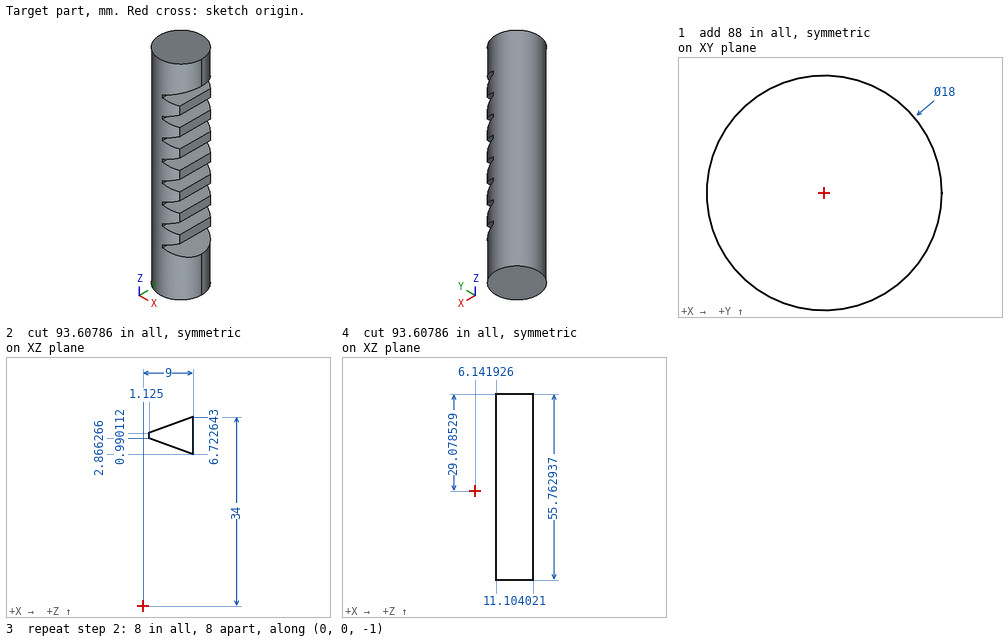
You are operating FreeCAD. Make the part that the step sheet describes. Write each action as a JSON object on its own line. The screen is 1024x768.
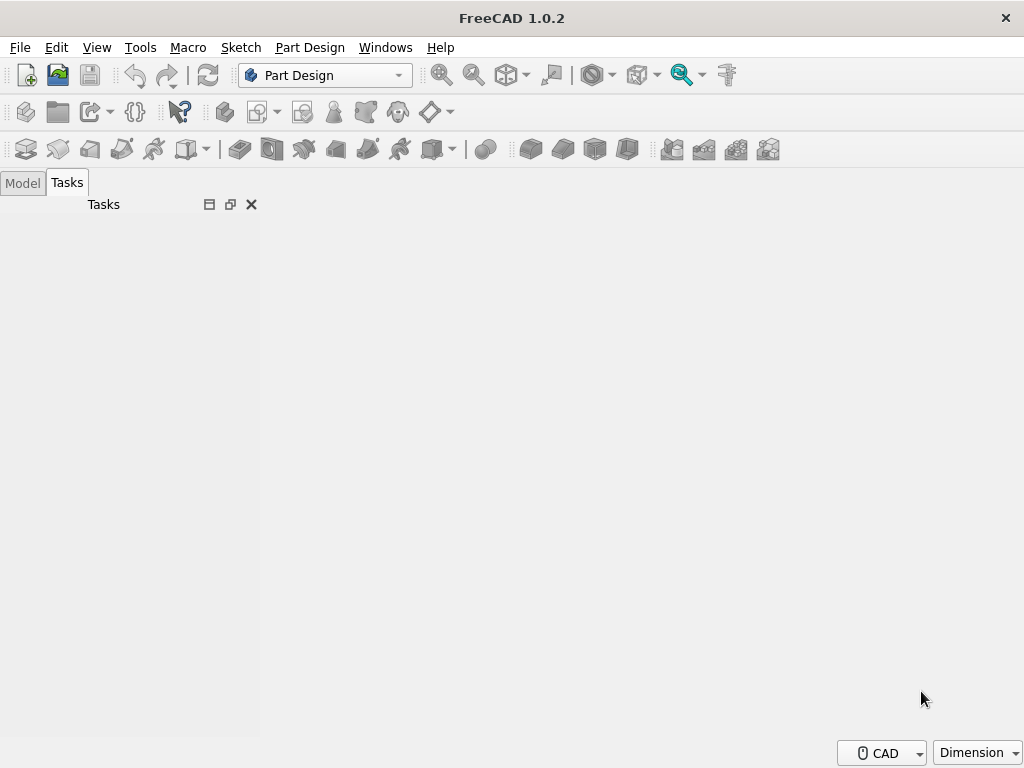
{"action": "left_click", "coordinate": [26, 76]}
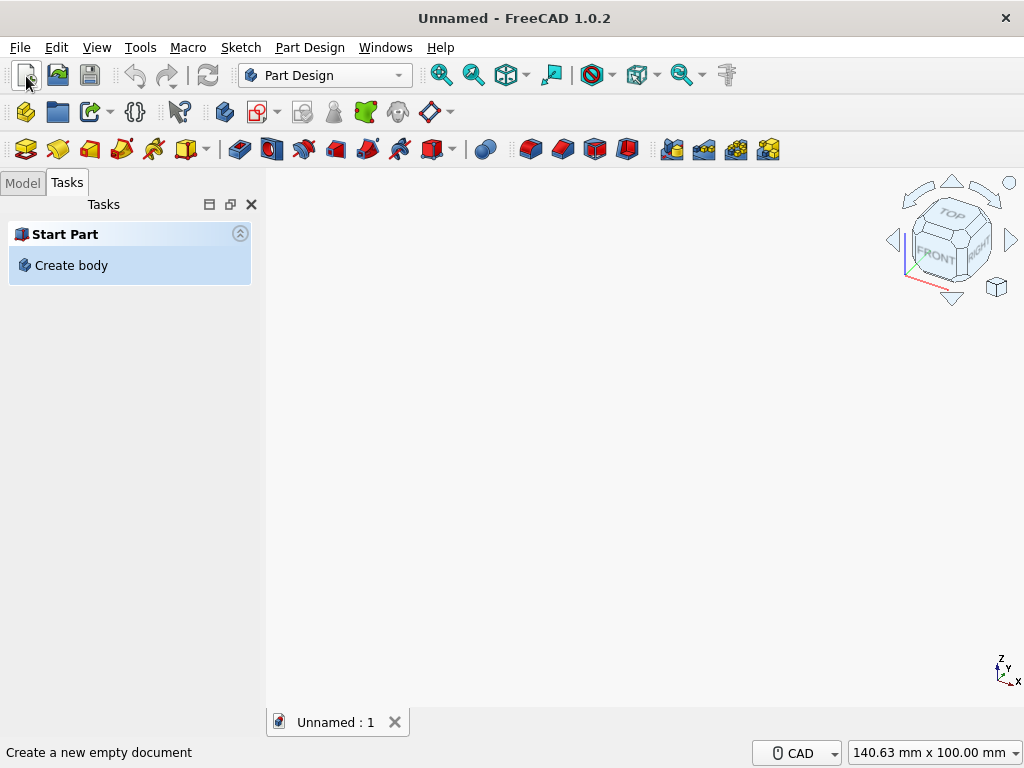
{"action": "left_click", "coordinate": [258, 112]}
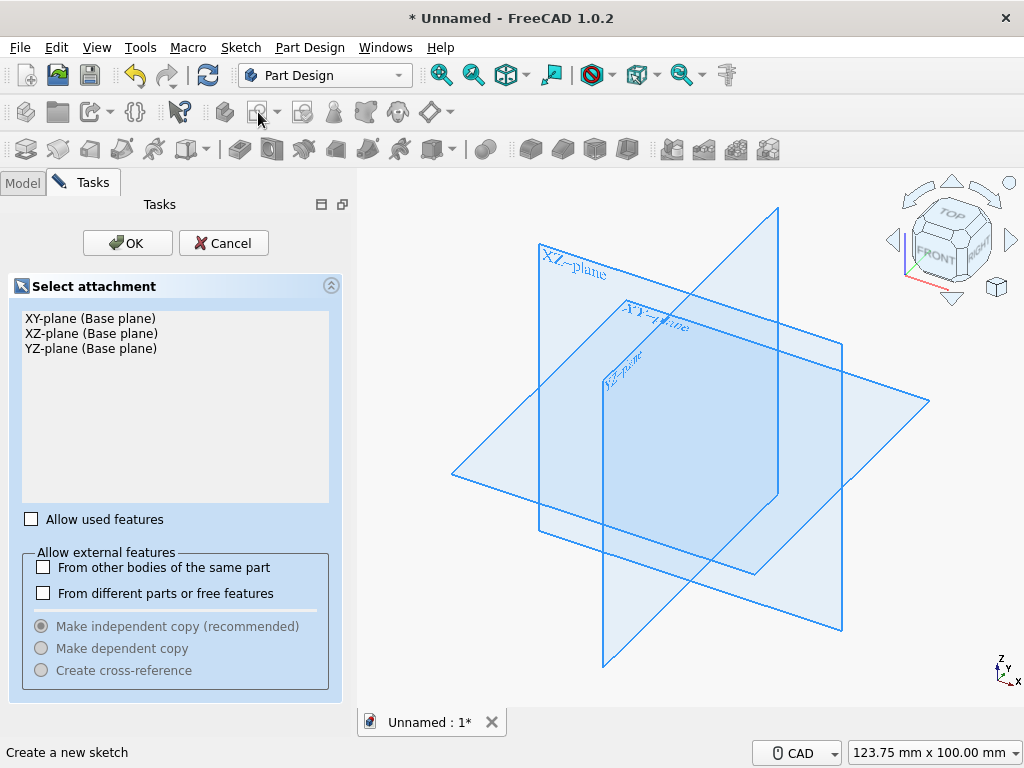
{"action": "left_click", "coordinate": [82, 318]}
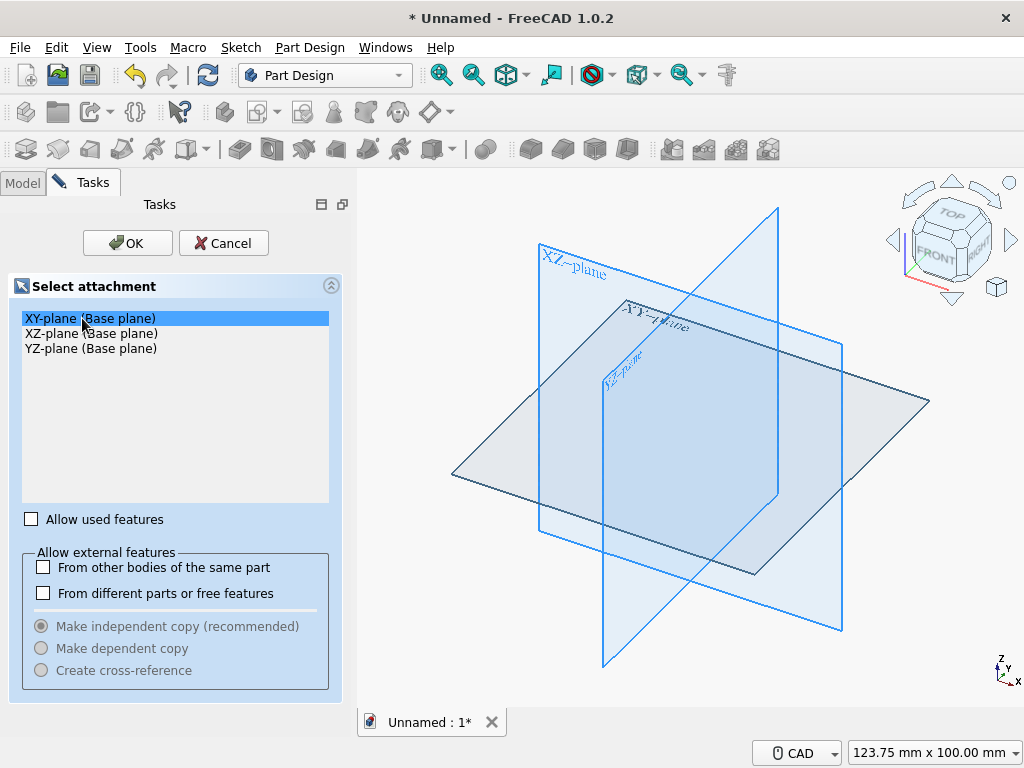
{"action": "left_click", "coordinate": [128, 243]}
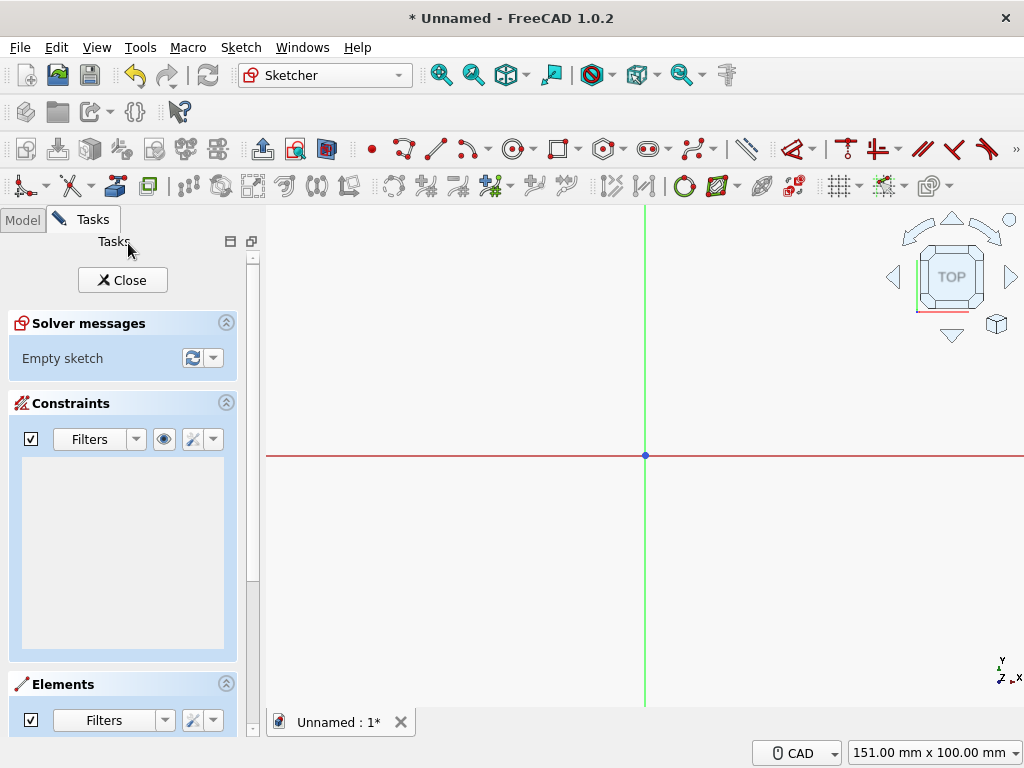
{"action": "scroll", "coordinate": [675, 456], "scroll_direction": "up", "scroll_amount": 6}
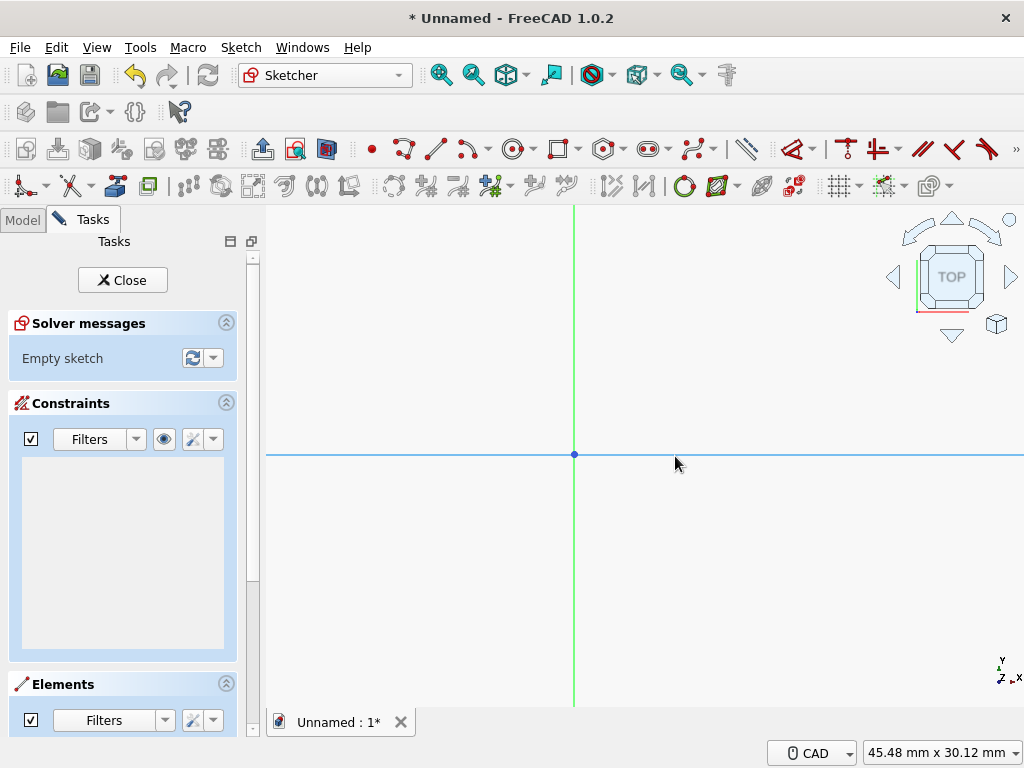
{"action": "left_click", "coordinate": [514, 150]}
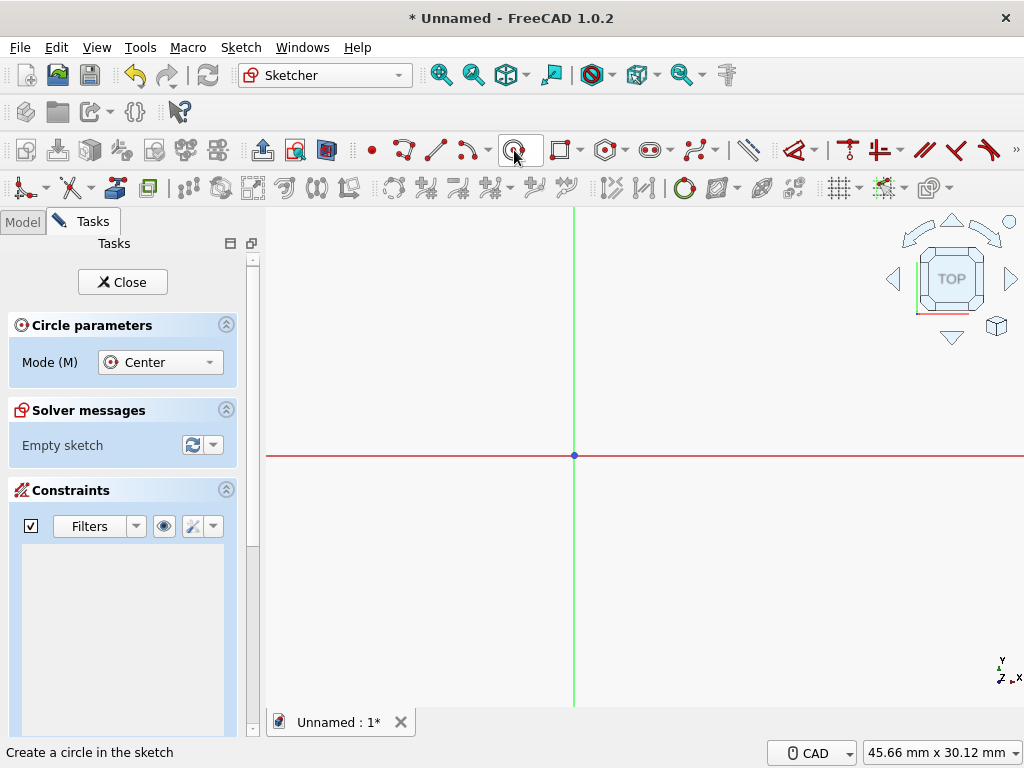
{"action": "left_click", "coordinate": [574, 456]}
{"action": "mouse_move", "coordinate": [680, 350]}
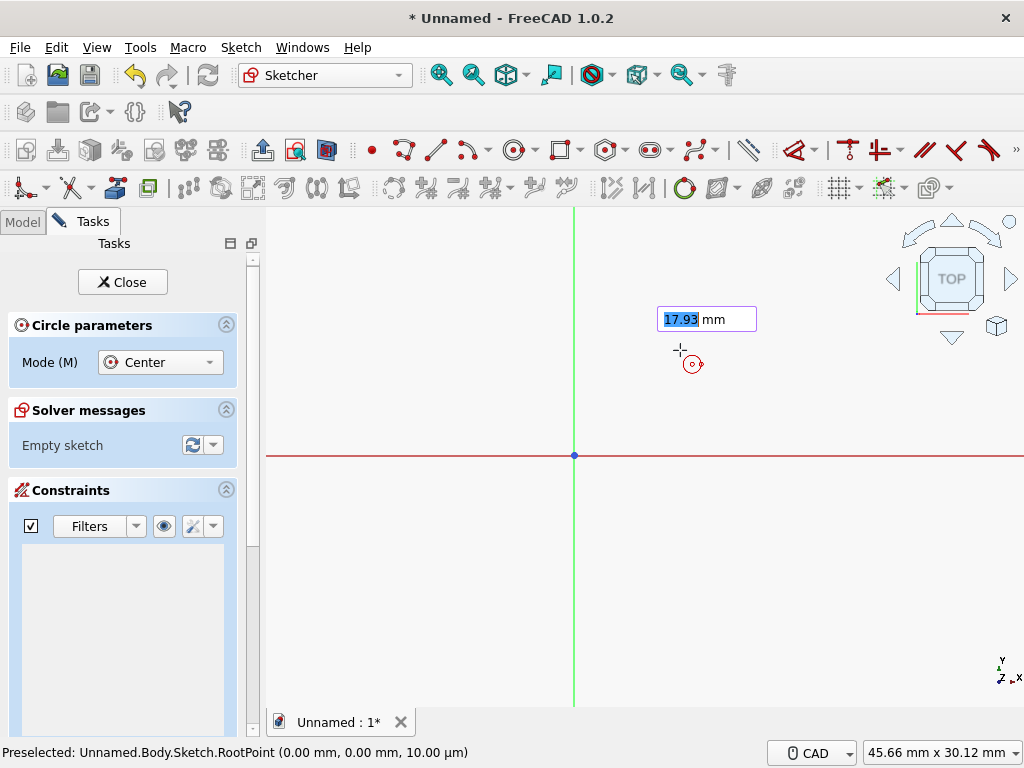
{"action": "type", "text": "18"}
{"action": "key", "text": "Return"}
{"action": "key", "text": "Escape"}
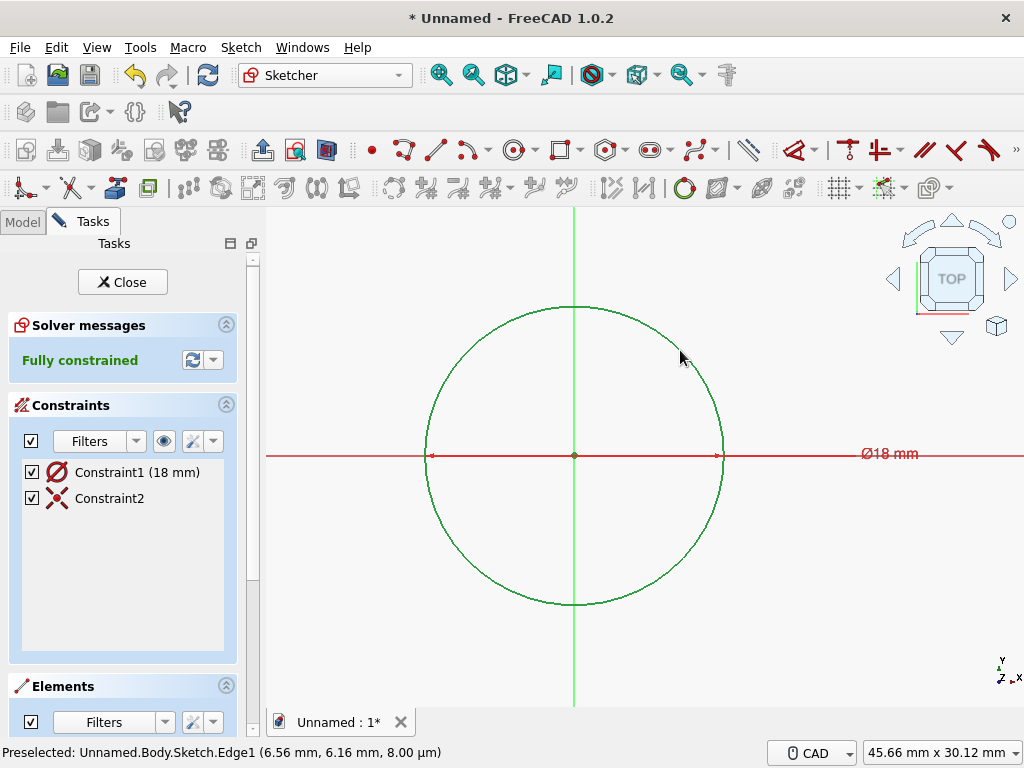
{"action": "left_click", "coordinate": [123, 282]}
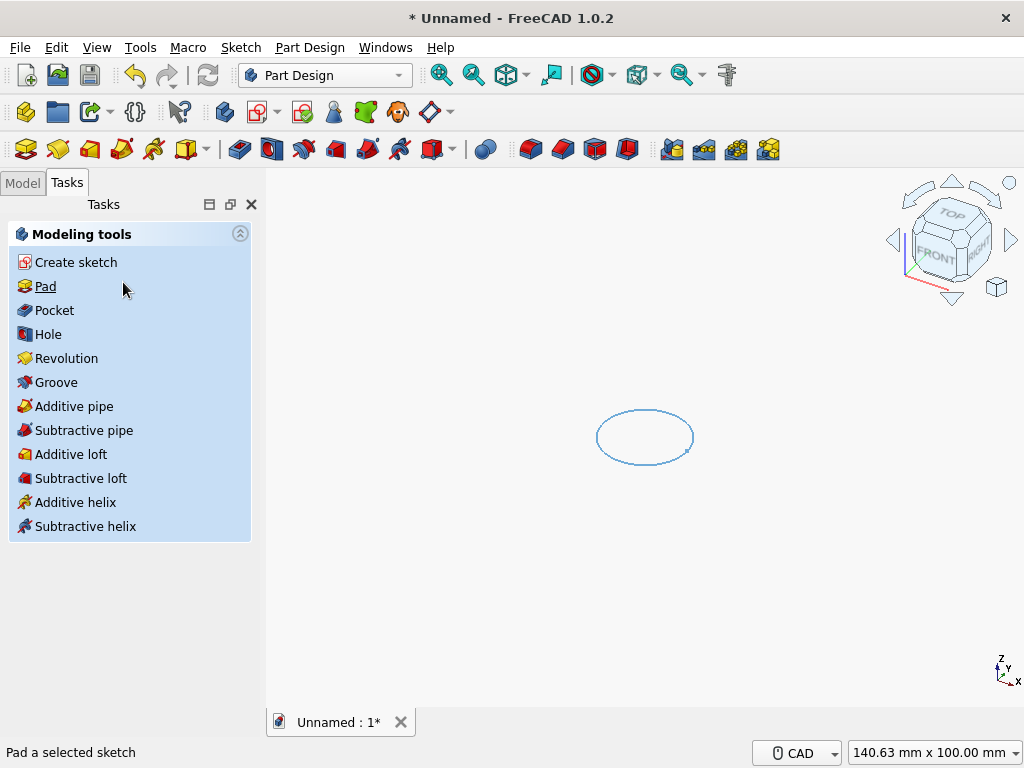
{"action": "left_click", "coordinate": [26, 150]}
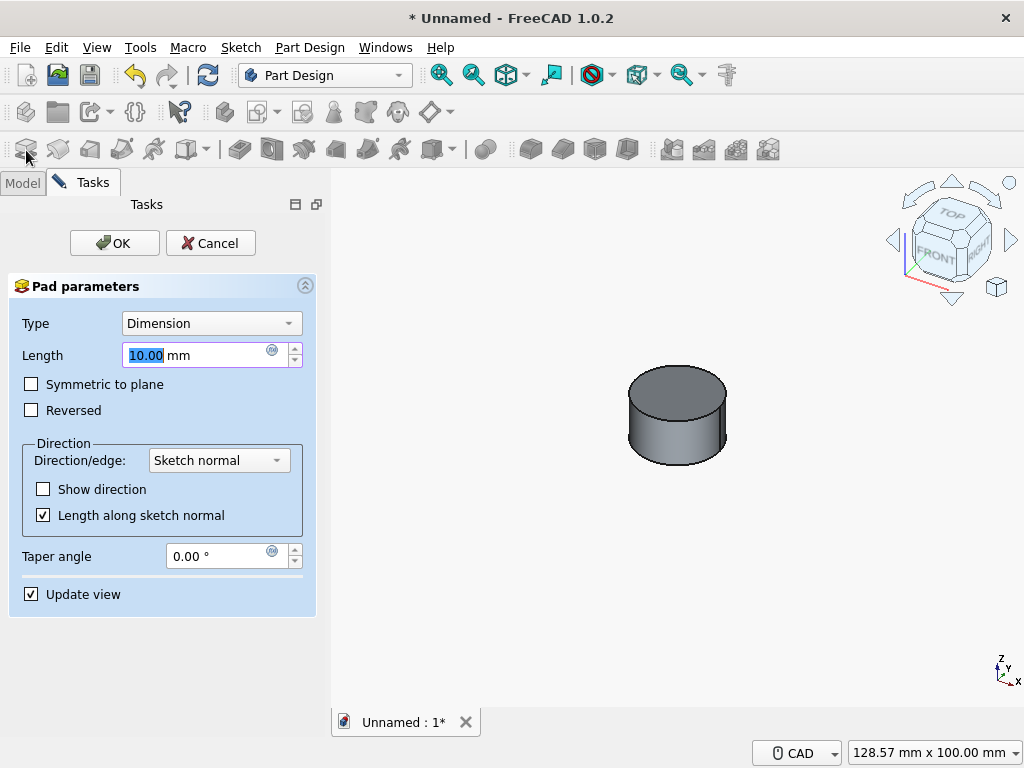
{"action": "type", "text": "88"}
{"action": "key", "text": "Tab"}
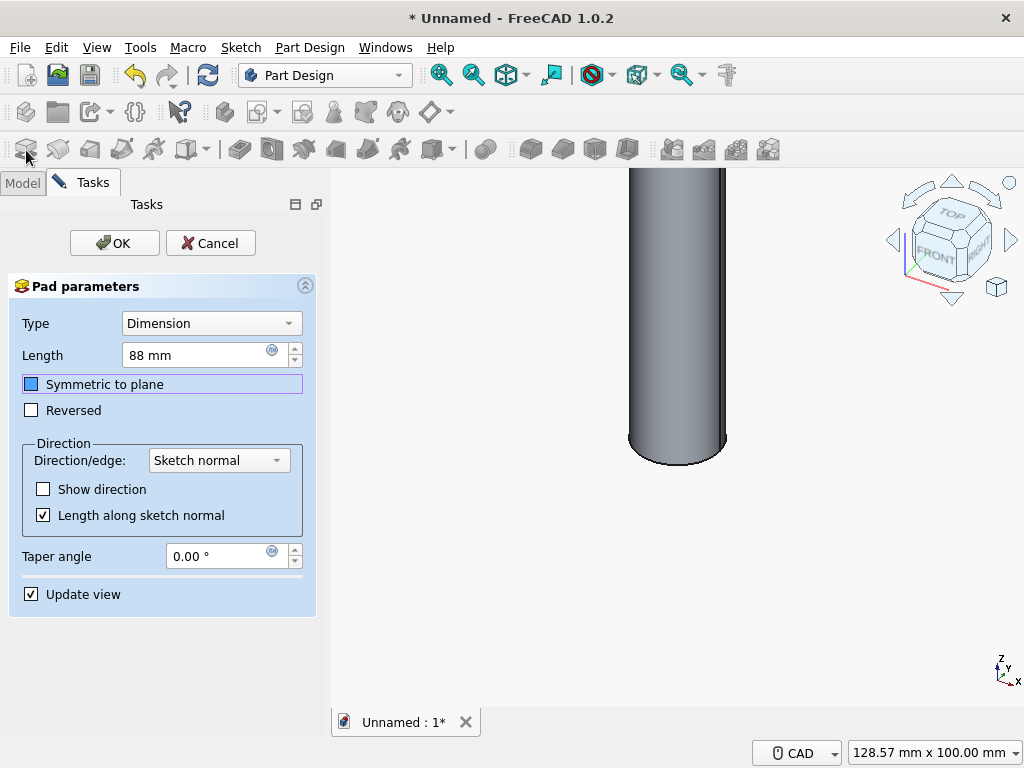
{"action": "left_click", "coordinate": [30, 384]}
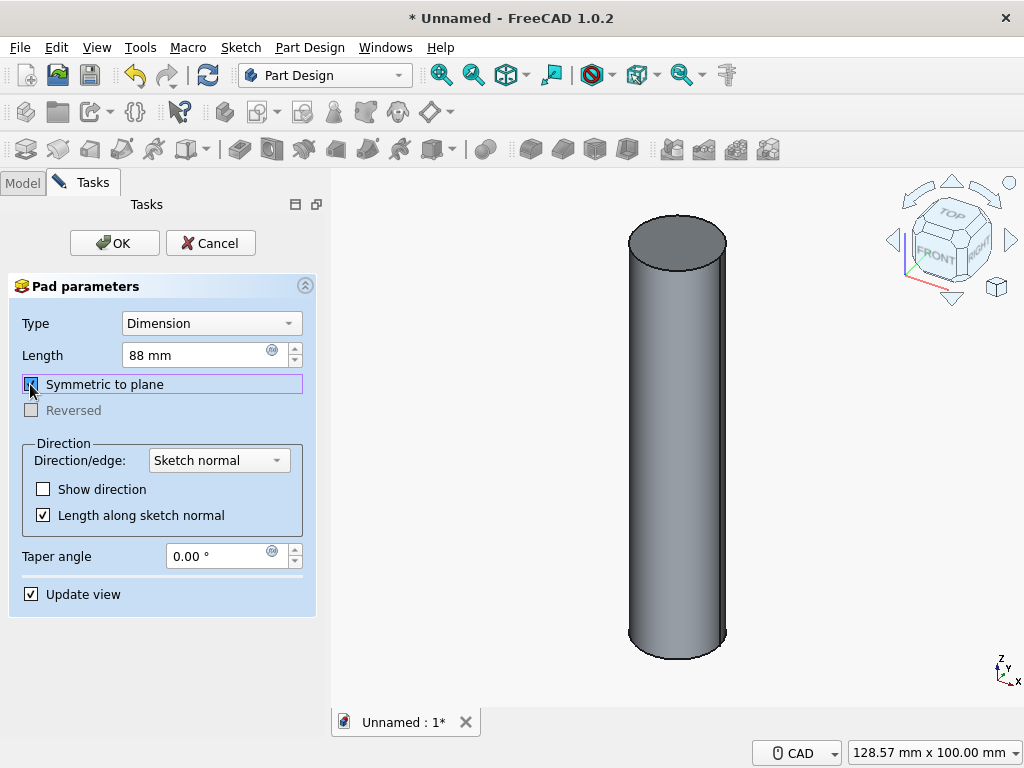
{"action": "left_click", "coordinate": [115, 243]}